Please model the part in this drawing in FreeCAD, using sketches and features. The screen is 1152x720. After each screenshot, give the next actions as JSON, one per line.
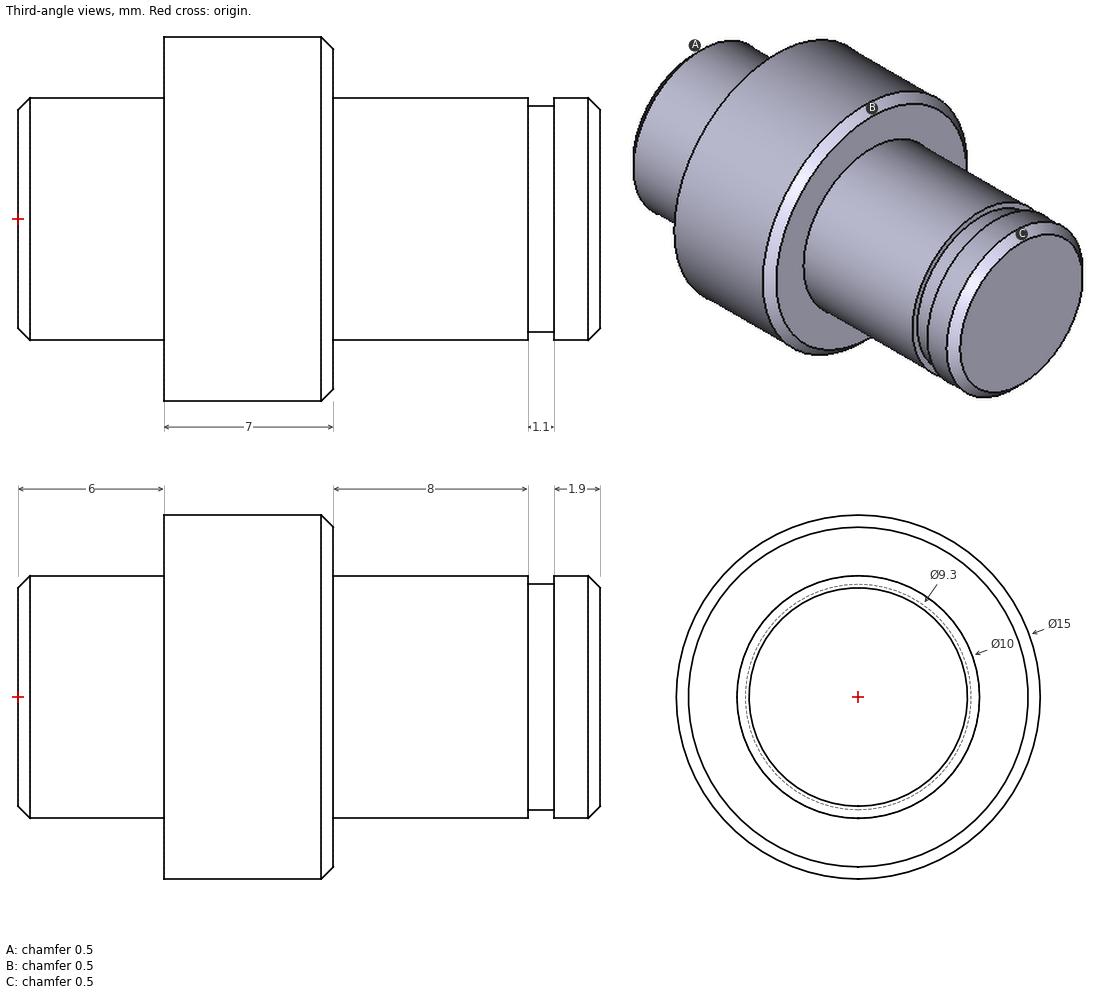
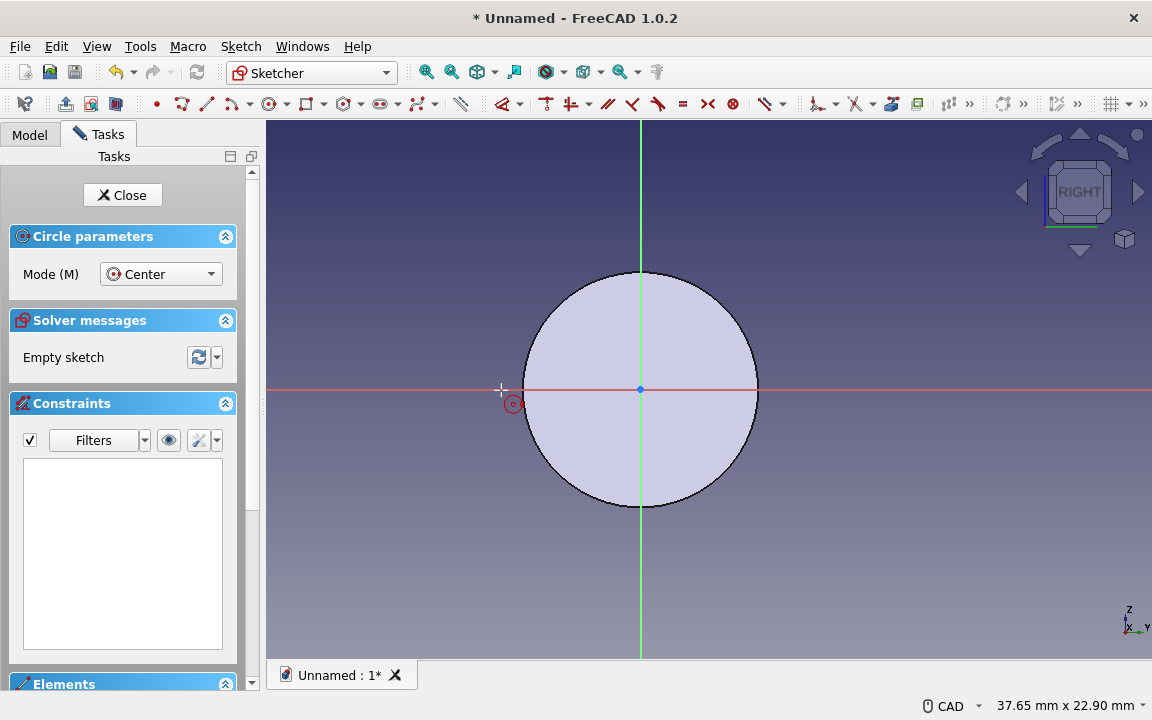
{"action": "left_click", "coordinate": [641, 390]}
{"action": "mouse_move", "coordinate": [765, 265]}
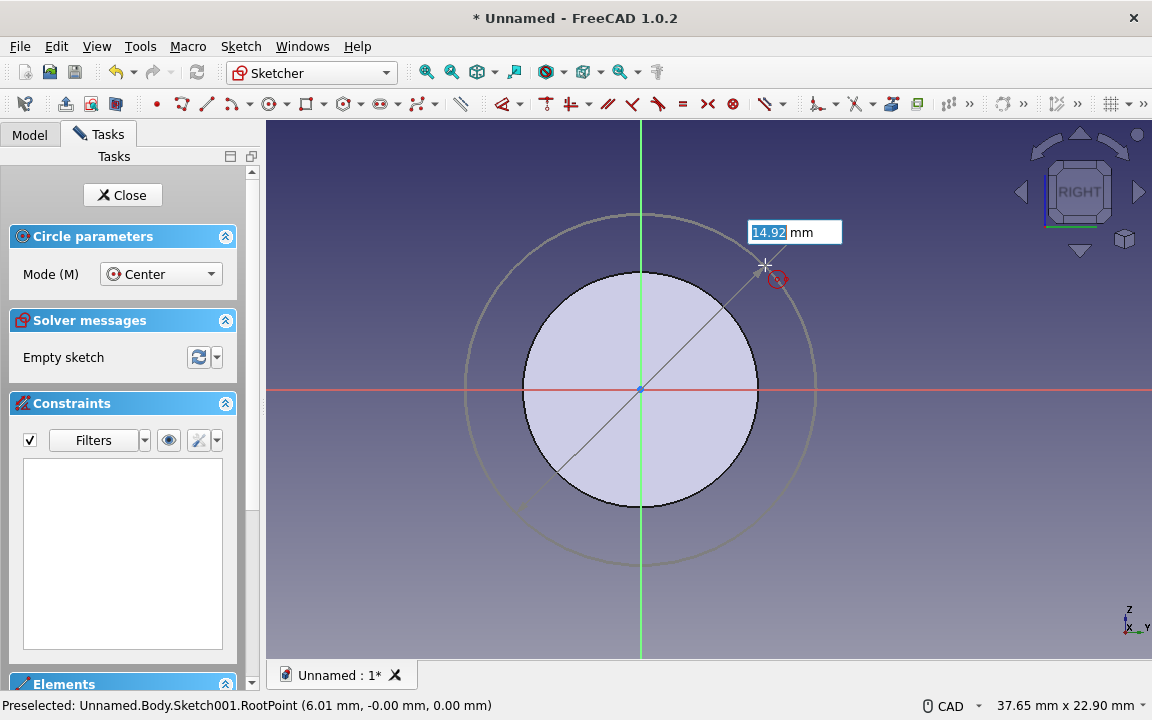
{"action": "type", "text": "15"}
{"action": "key", "text": "Return"}
{"action": "key", "text": "Escape"}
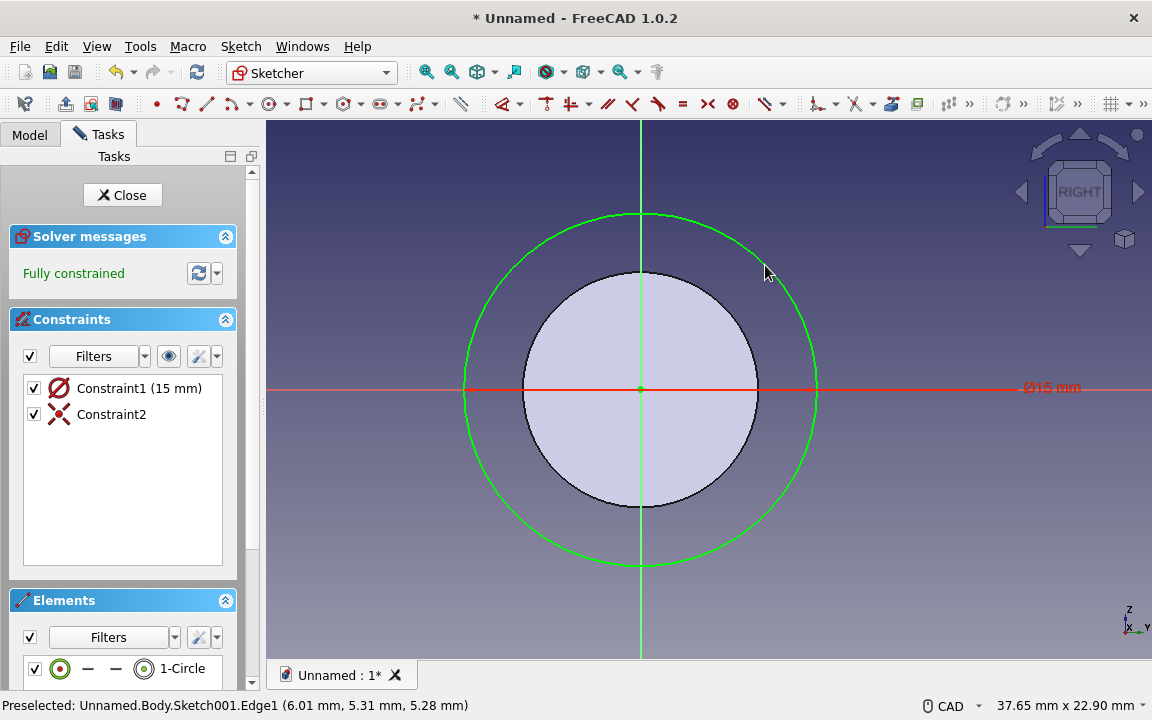
{"action": "left_click", "coordinate": [123, 195]}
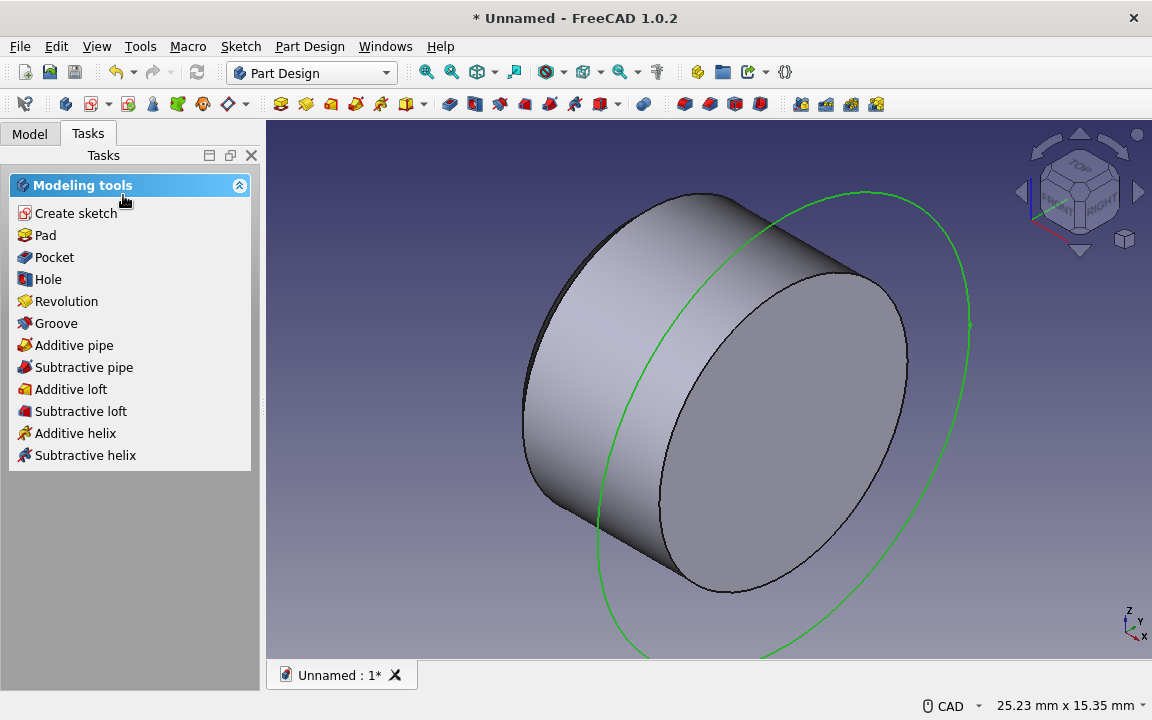
{"action": "left_click", "coordinate": [281, 104]}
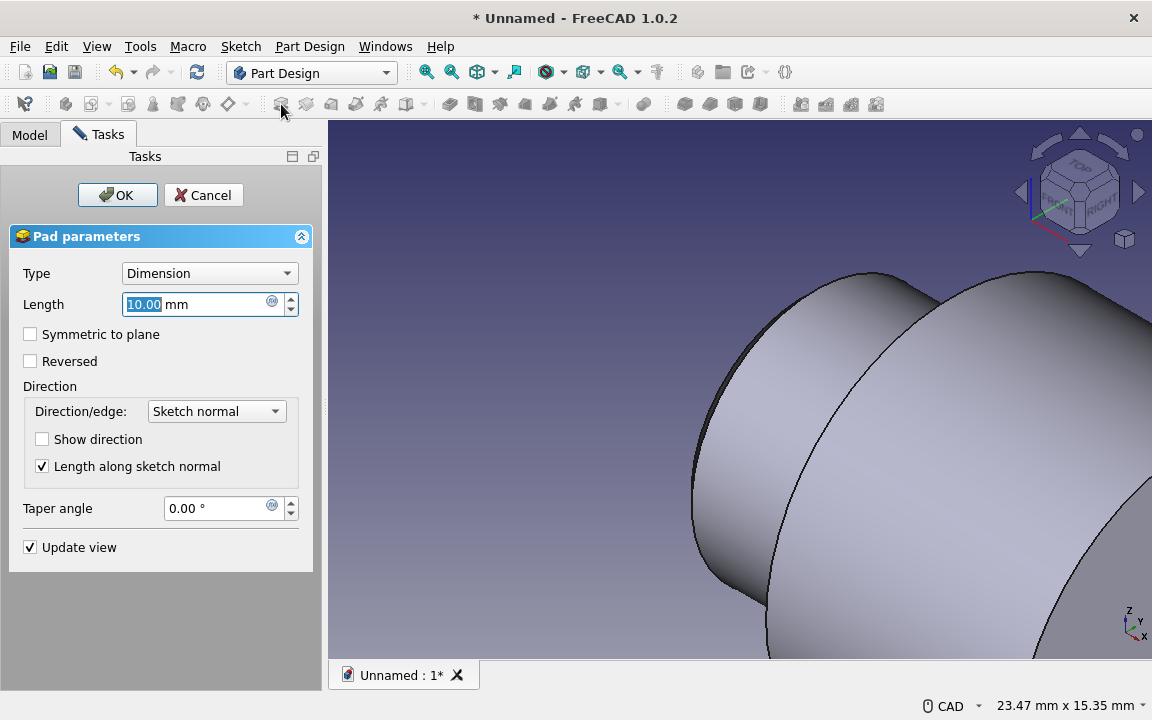
{"action": "type", "text": "7"}
{"action": "key", "text": "Tab"}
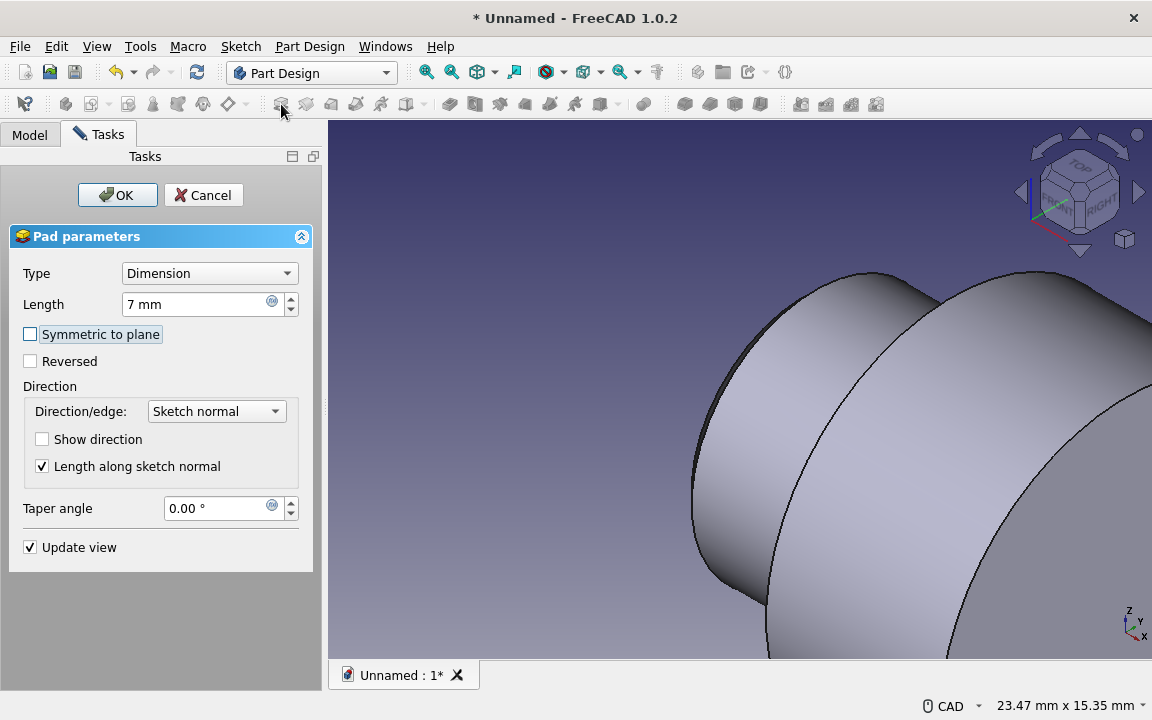
{"action": "left_click", "coordinate": [118, 195]}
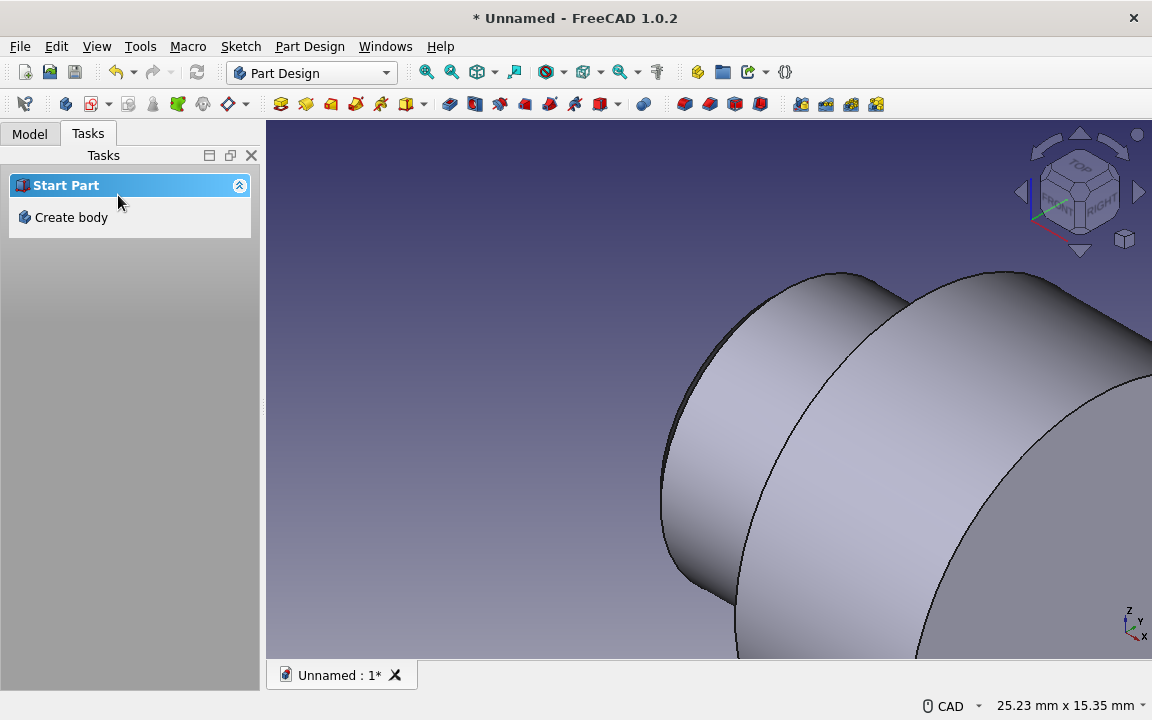
{"action": "key", "text": "v f"}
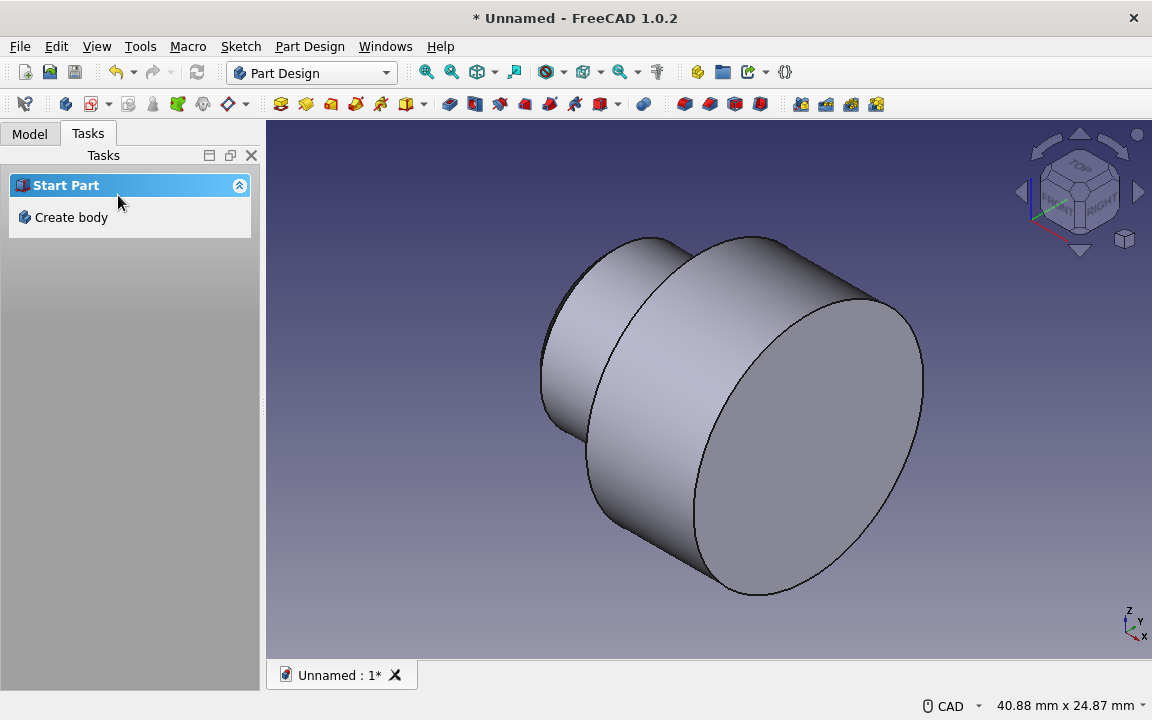
{"action": "left_click", "coordinate": [694, 512]}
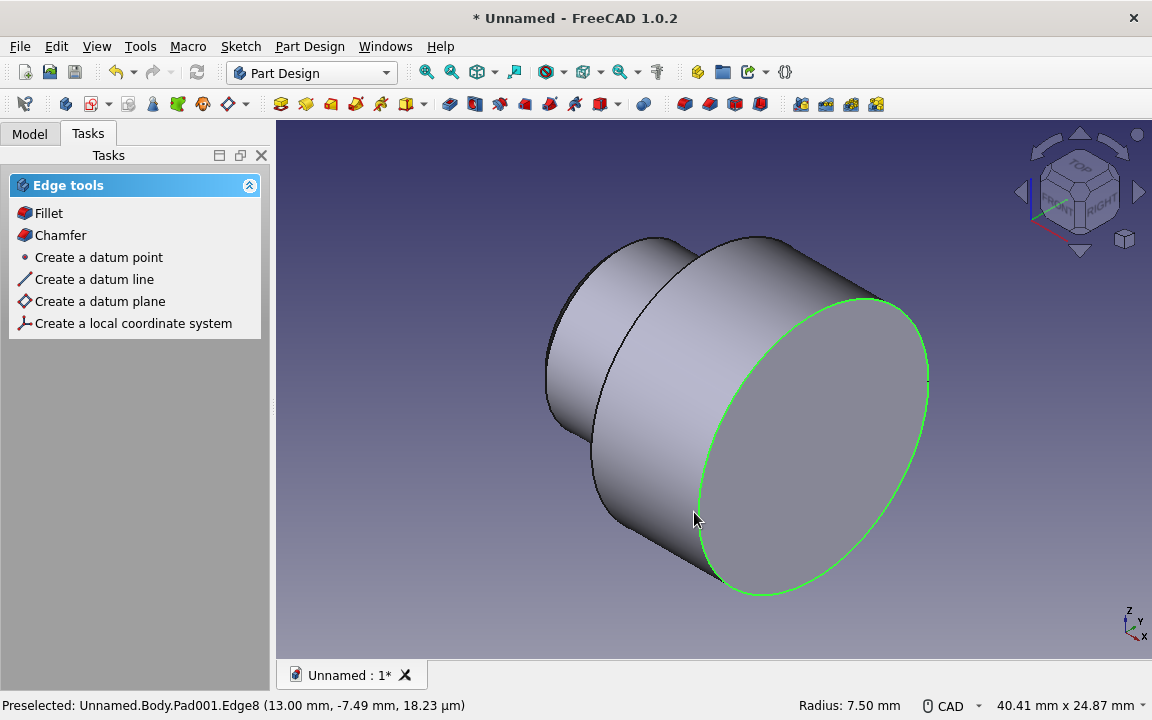
{"action": "left_click", "coordinate": [710, 104]}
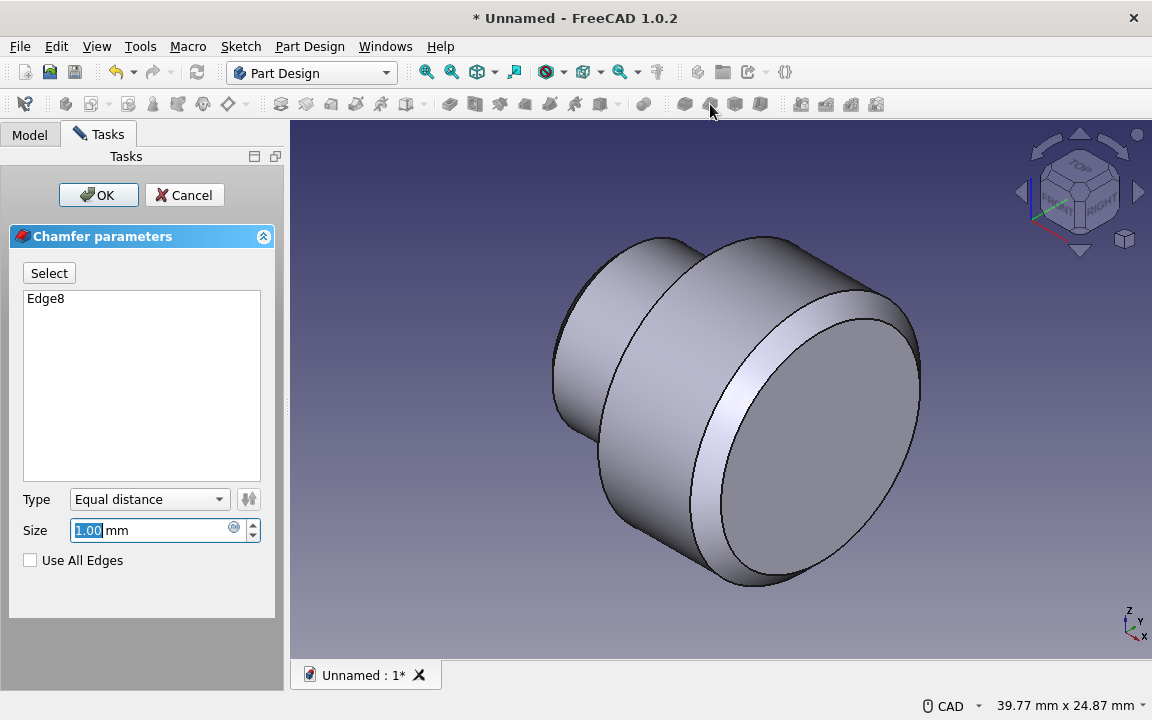
{"action": "type", "text": "0.5"}
{"action": "key", "text": "Tab"}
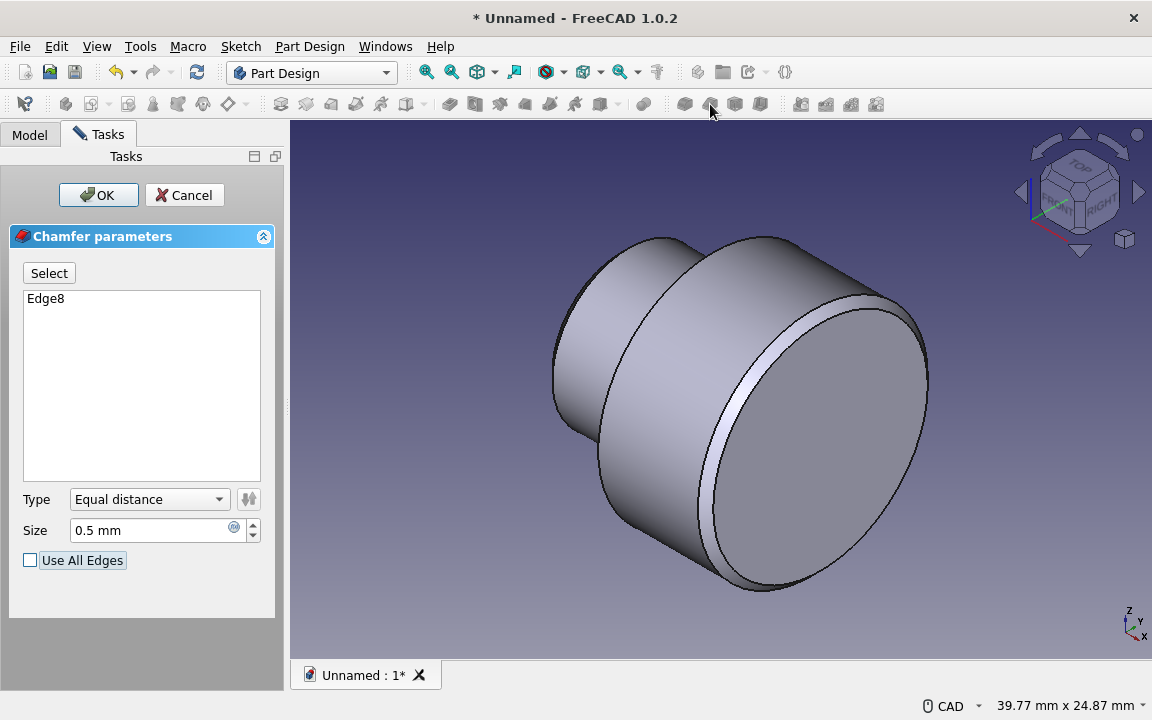
{"action": "left_click", "coordinate": [99, 195]}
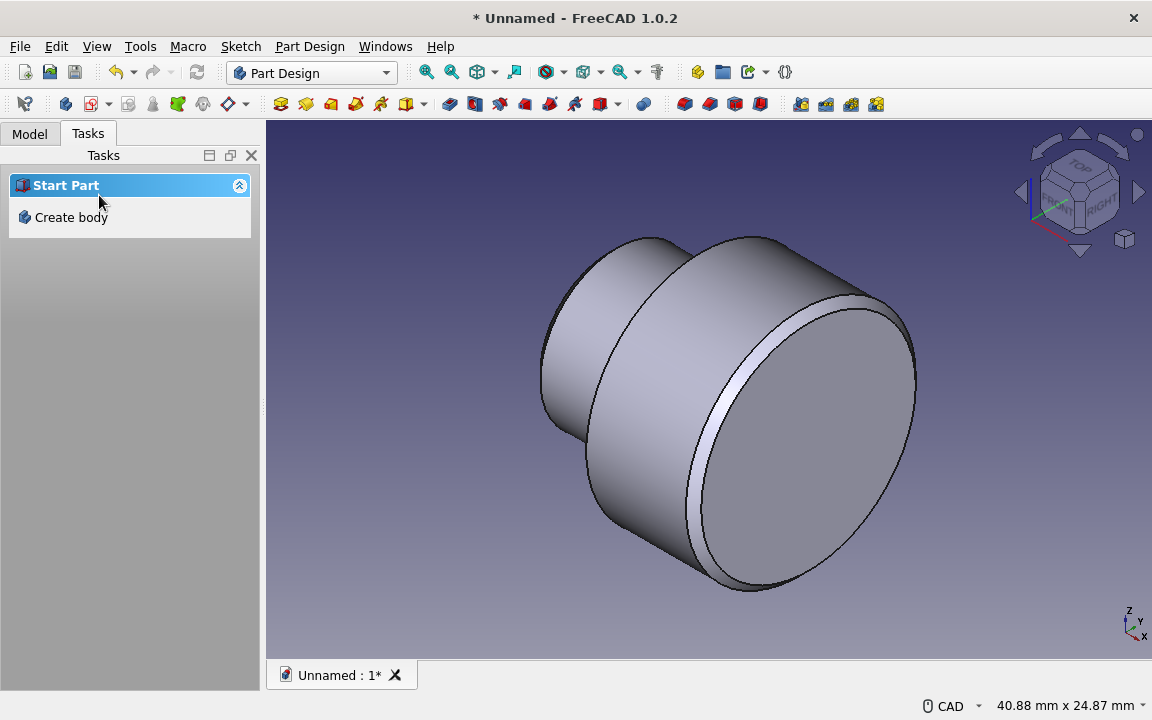
{"action": "left_click", "coordinate": [809, 446]}